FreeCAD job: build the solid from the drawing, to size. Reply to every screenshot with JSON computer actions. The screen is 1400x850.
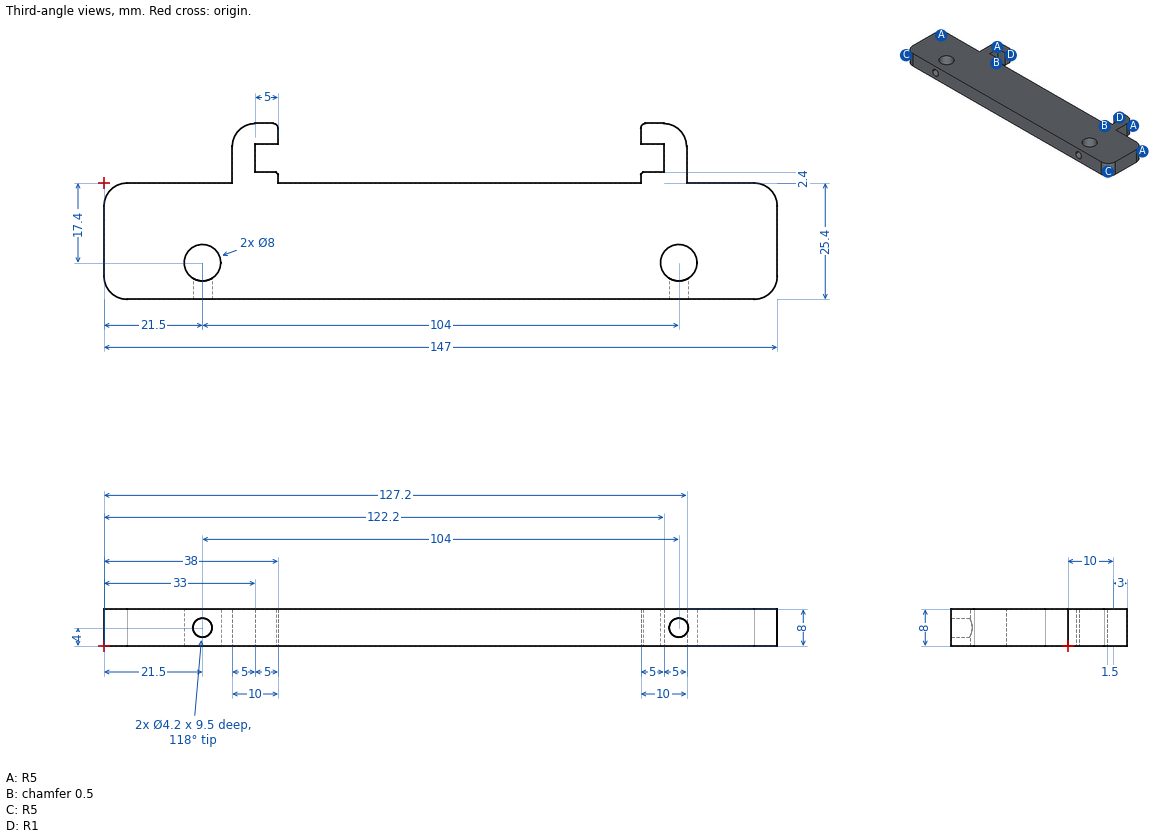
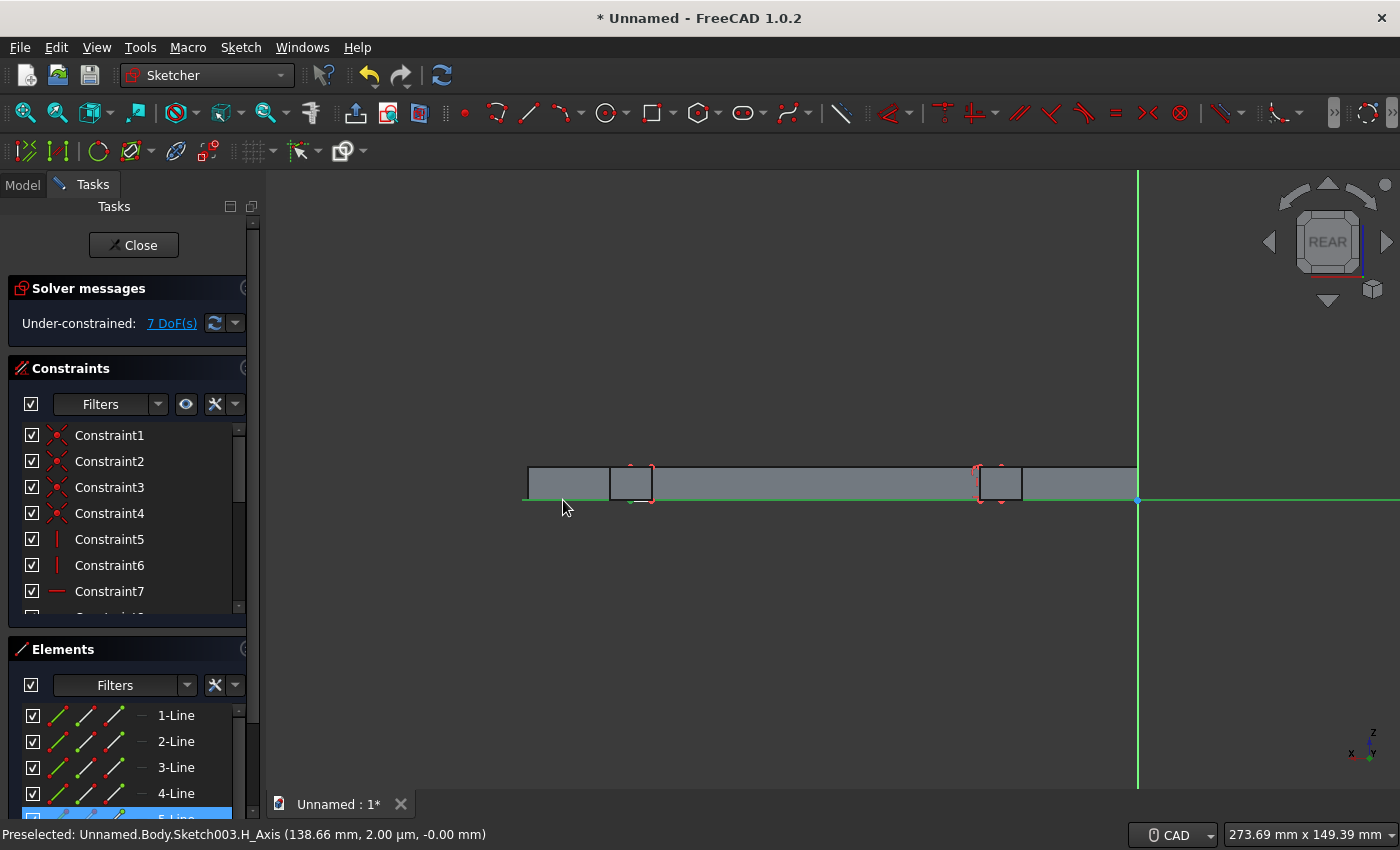
{"action": "left_click", "coordinate": [944, 114]}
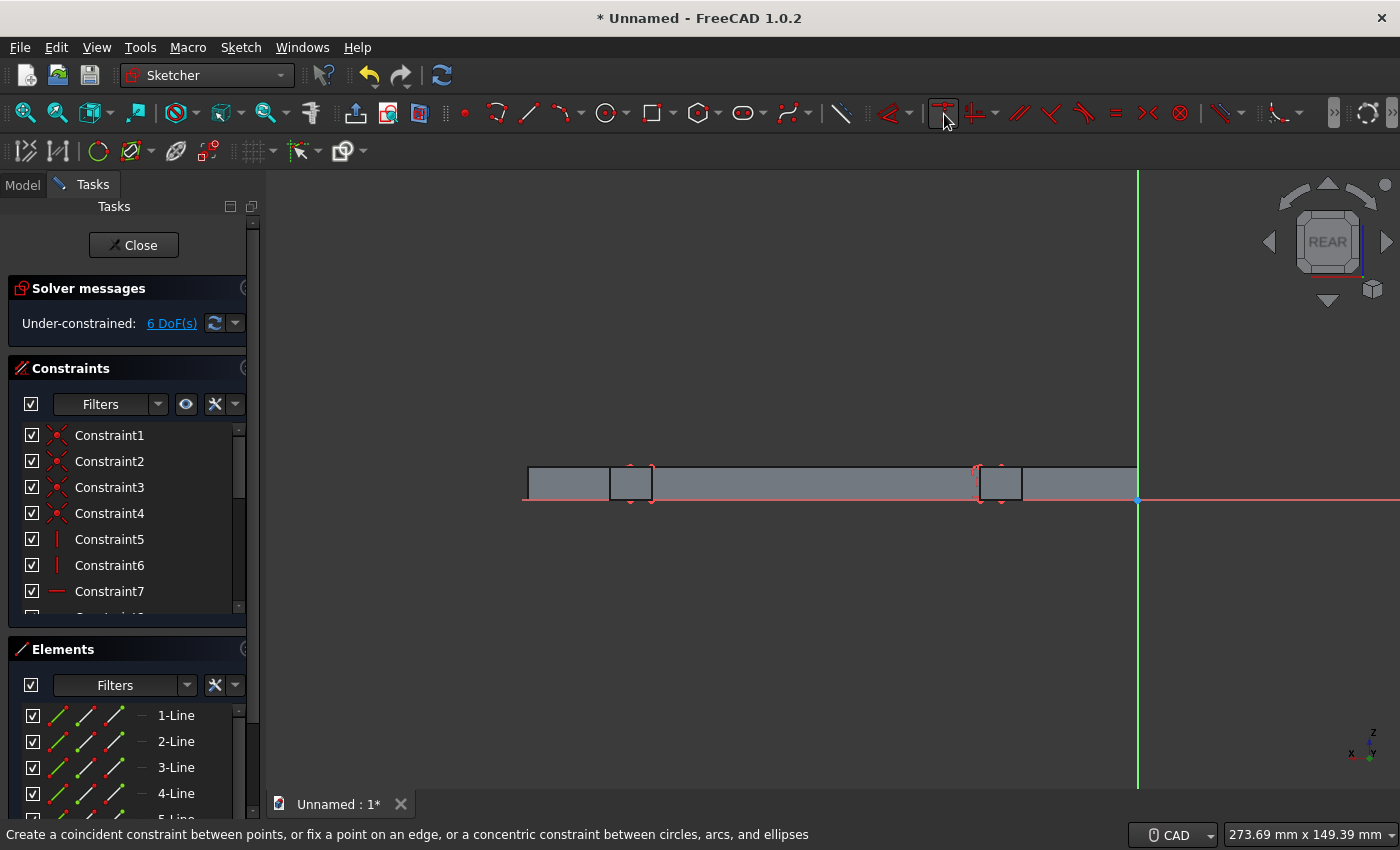
{"action": "left_click", "coordinate": [888, 114]}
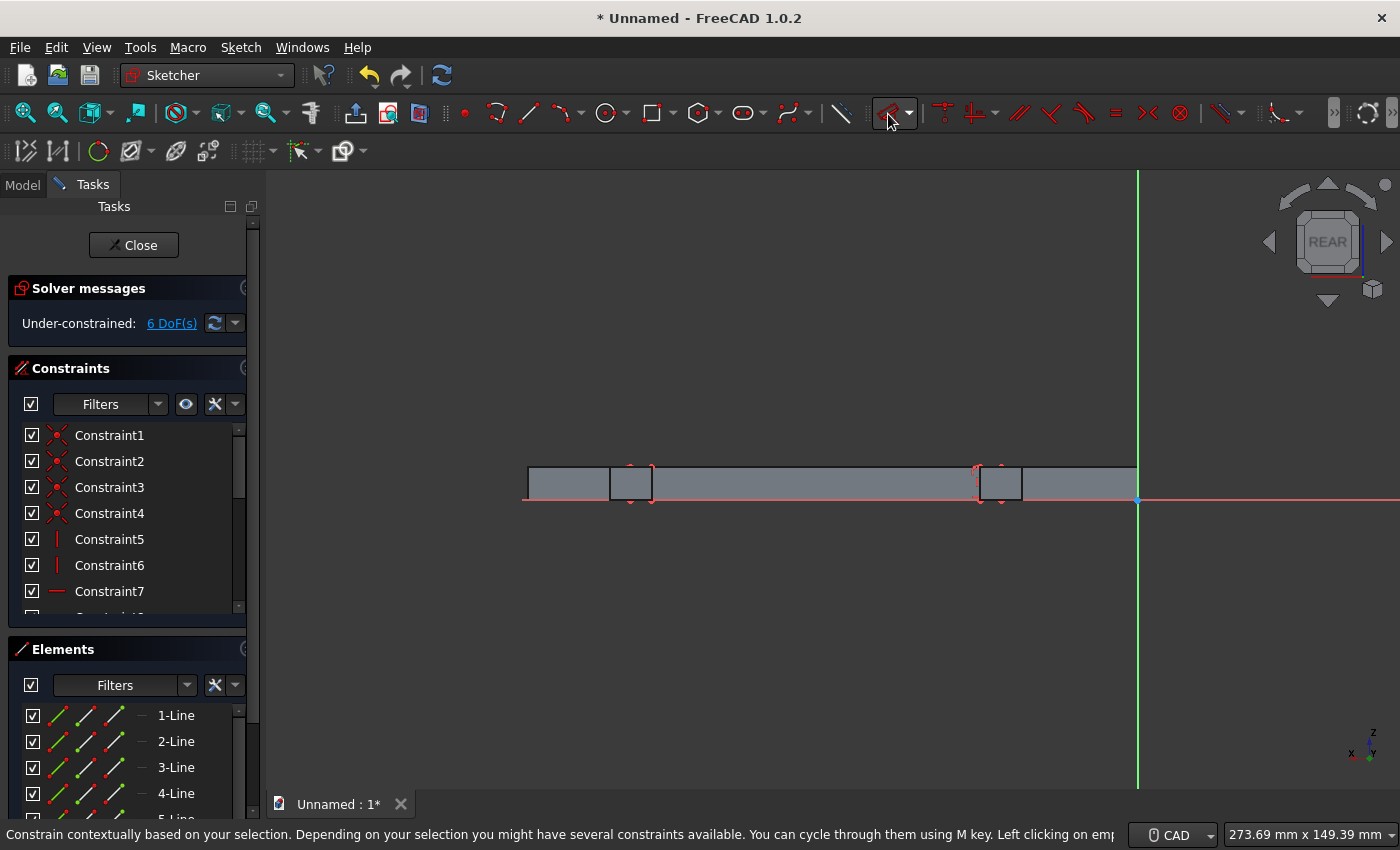
{"action": "scroll", "coordinate": [980, 478], "scroll_direction": "up", "scroll_amount": 2}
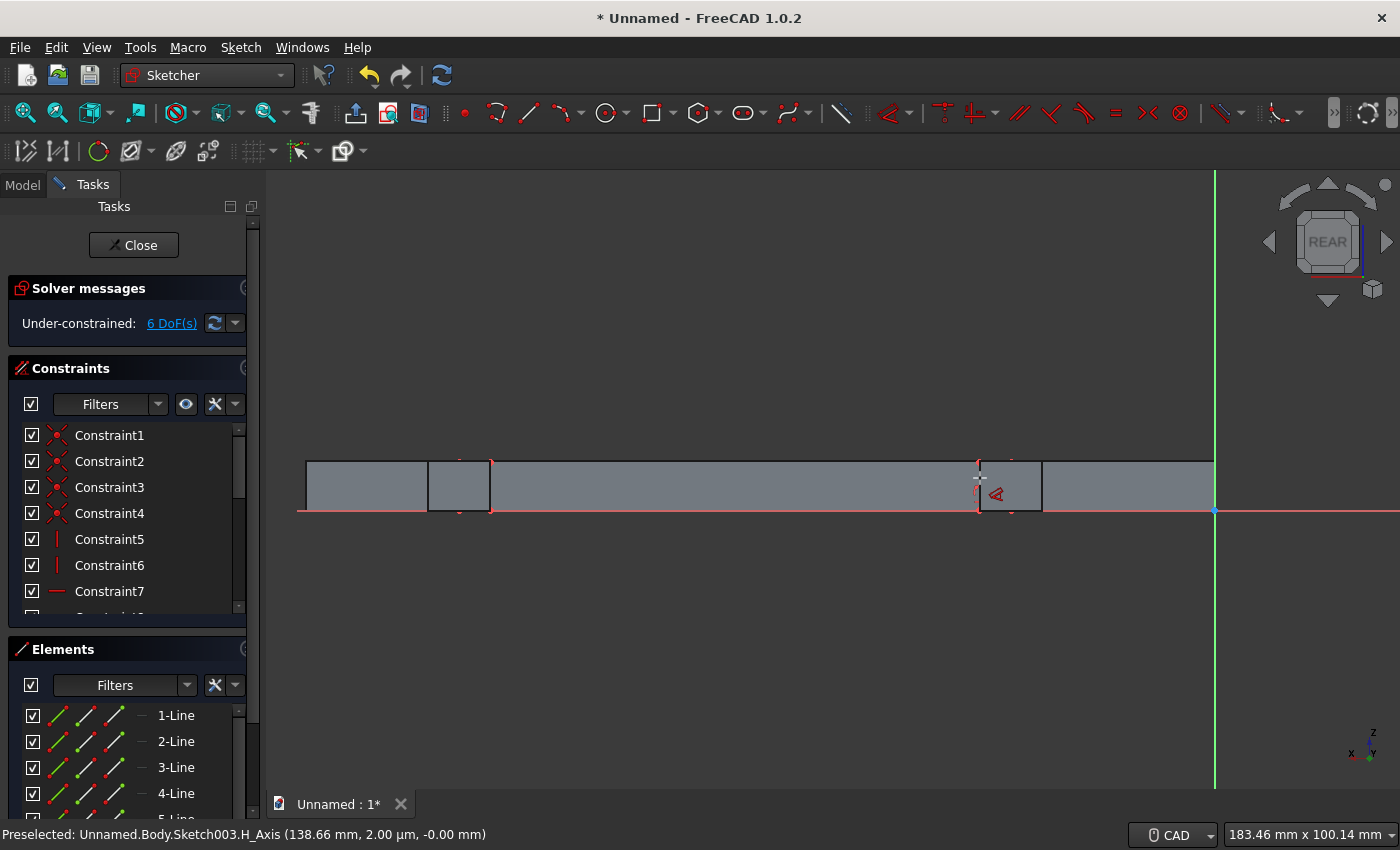
{"action": "left_click", "coordinate": [980, 477]}
{"action": "left_click", "coordinate": [946, 487]}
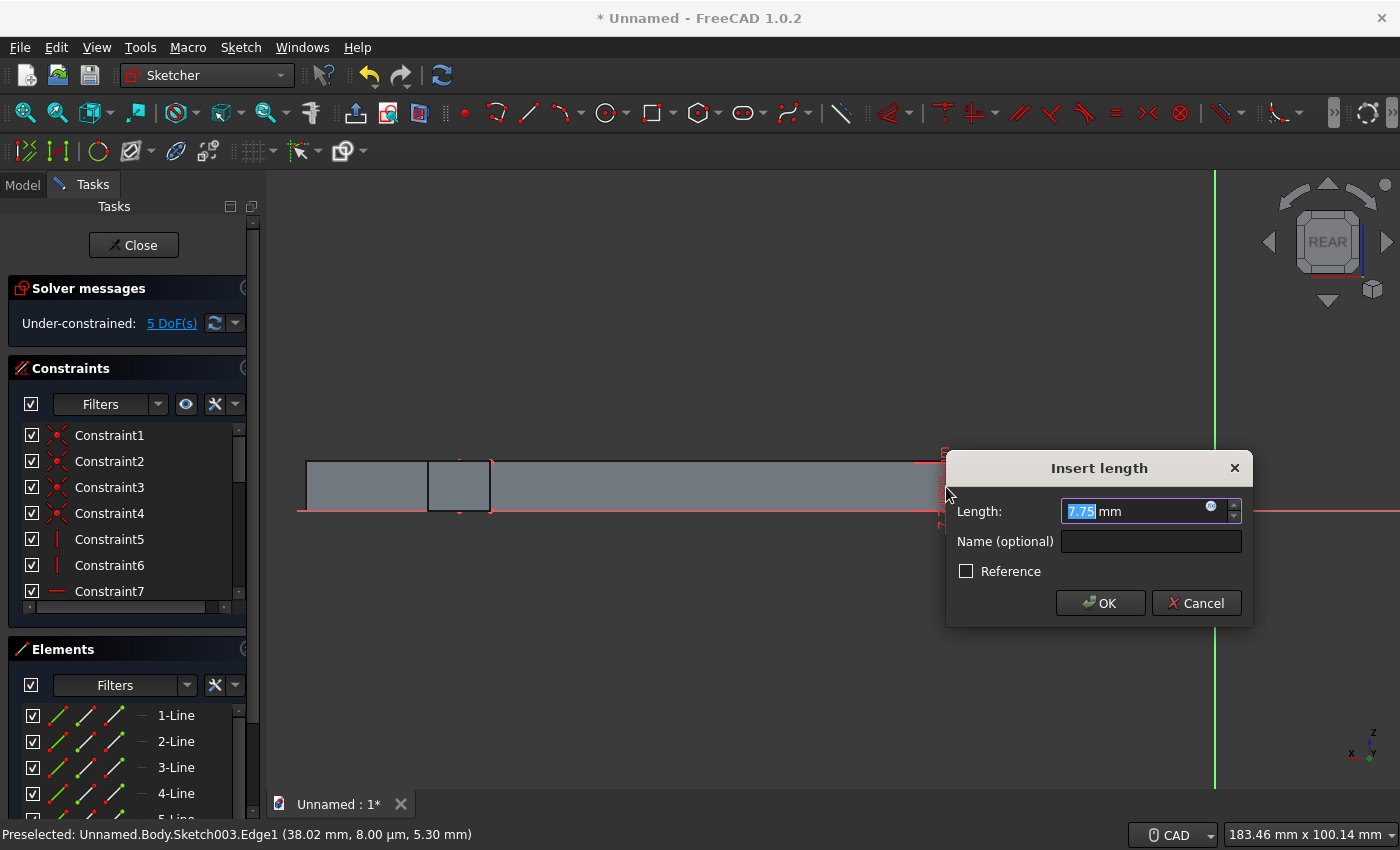
{"action": "type", "text": "8"}
{"action": "key", "text": "Return"}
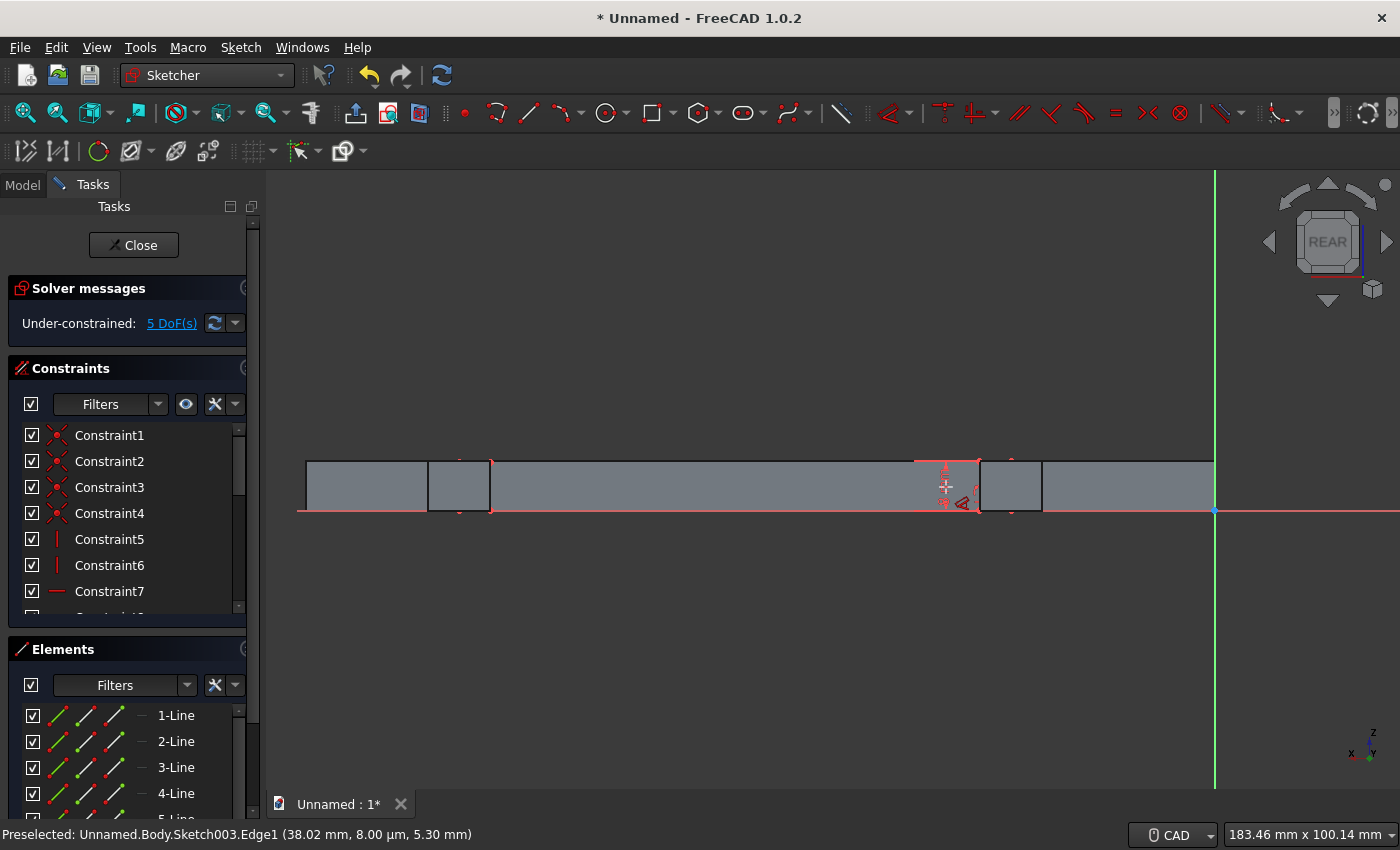
{"action": "scroll", "coordinate": [989, 511], "scroll_direction": "up", "scroll_amount": 2}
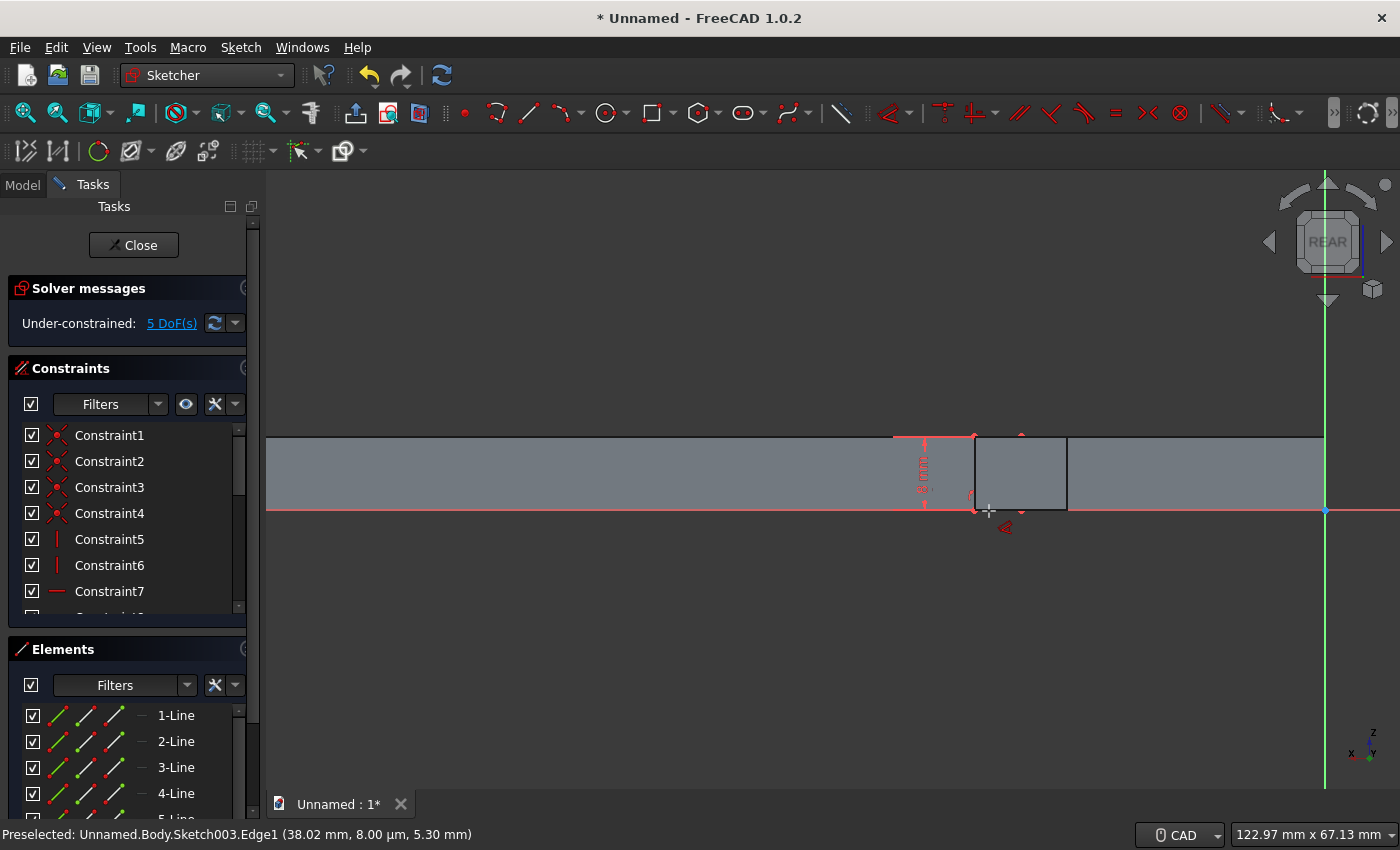
{"action": "left_click", "coordinate": [989, 510]}
{"action": "left_click", "coordinate": [998, 544]}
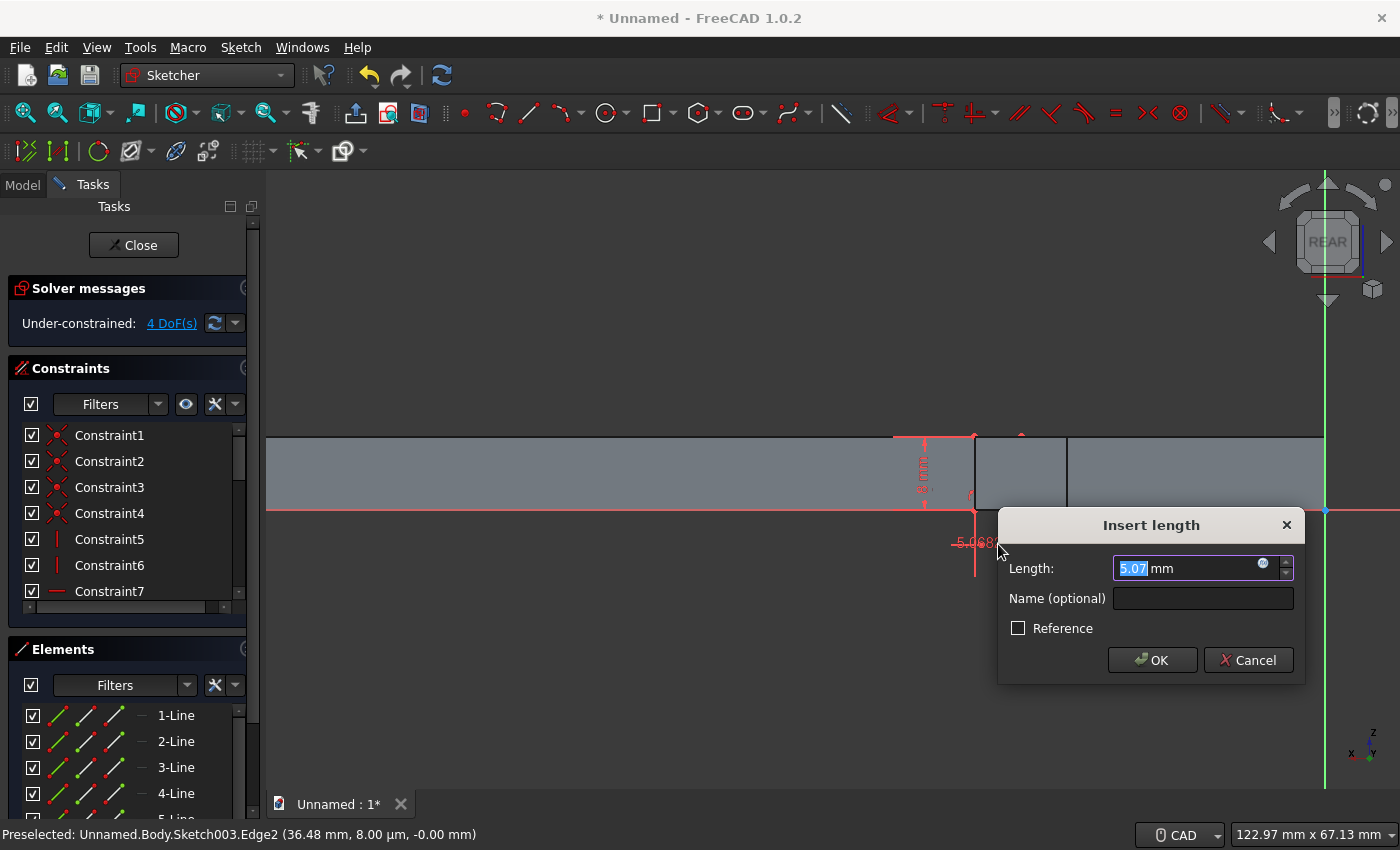
{"action": "type", "text": "5"}
{"action": "key", "text": "Return"}